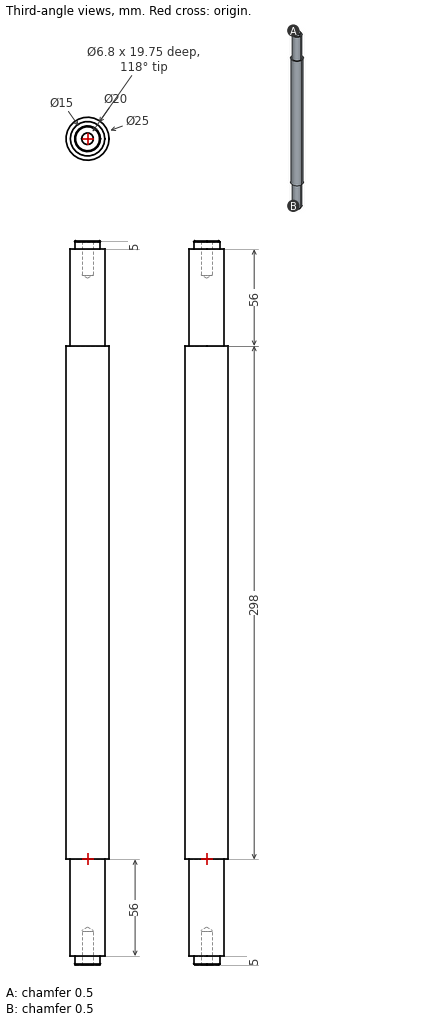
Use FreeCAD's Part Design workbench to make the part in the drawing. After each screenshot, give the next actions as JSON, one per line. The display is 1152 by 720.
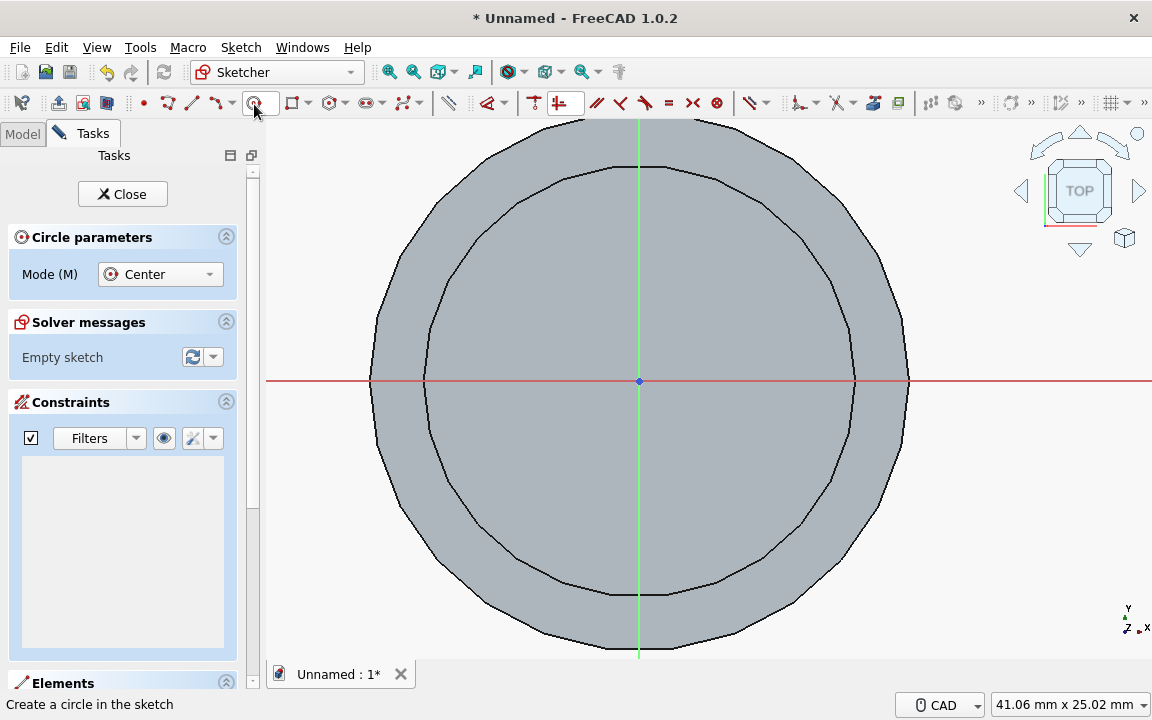
{"action": "left_click", "coordinate": [639, 381]}
{"action": "left_click", "coordinate": [754, 267]}
{"action": "key", "text": "Escape"}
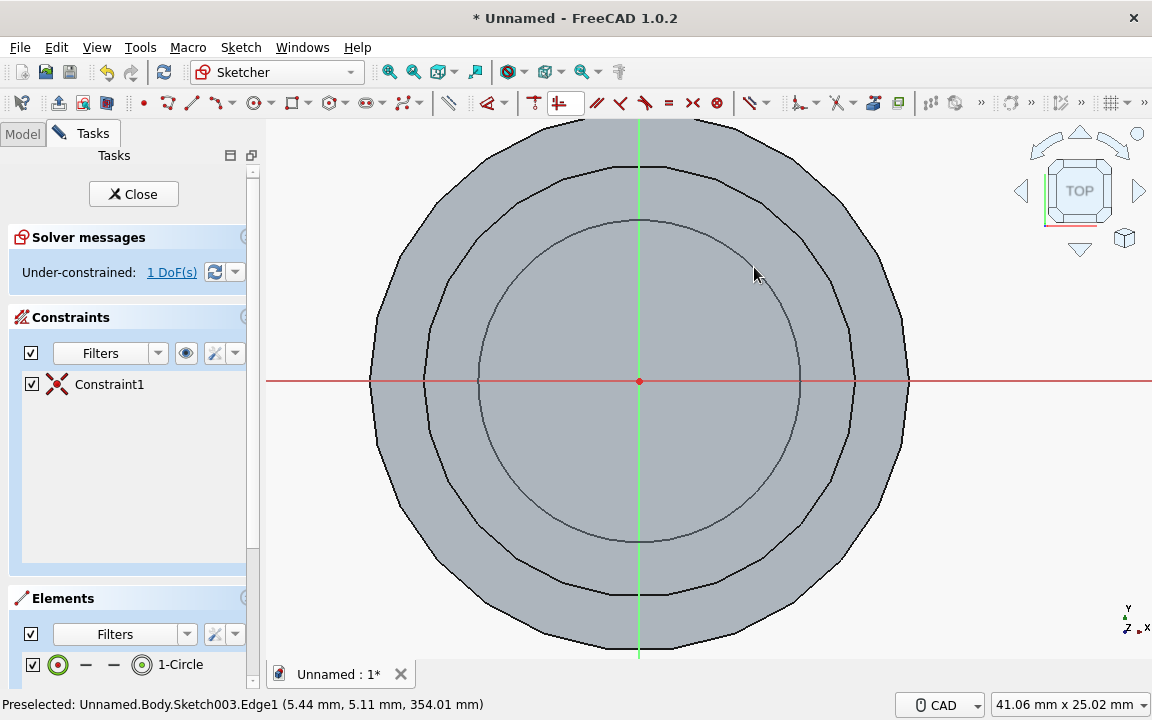
{"action": "left_click", "coordinate": [488, 104]}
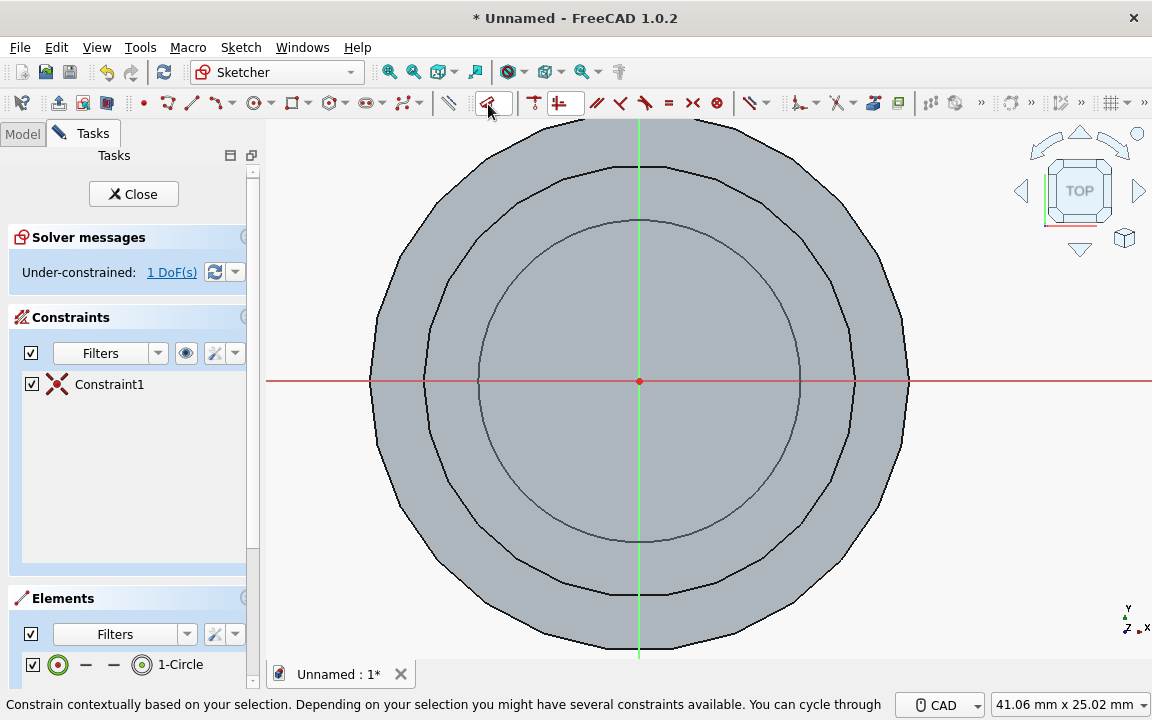
{"action": "left_click", "coordinate": [753, 267]}
{"action": "left_click", "coordinate": [776, 244]}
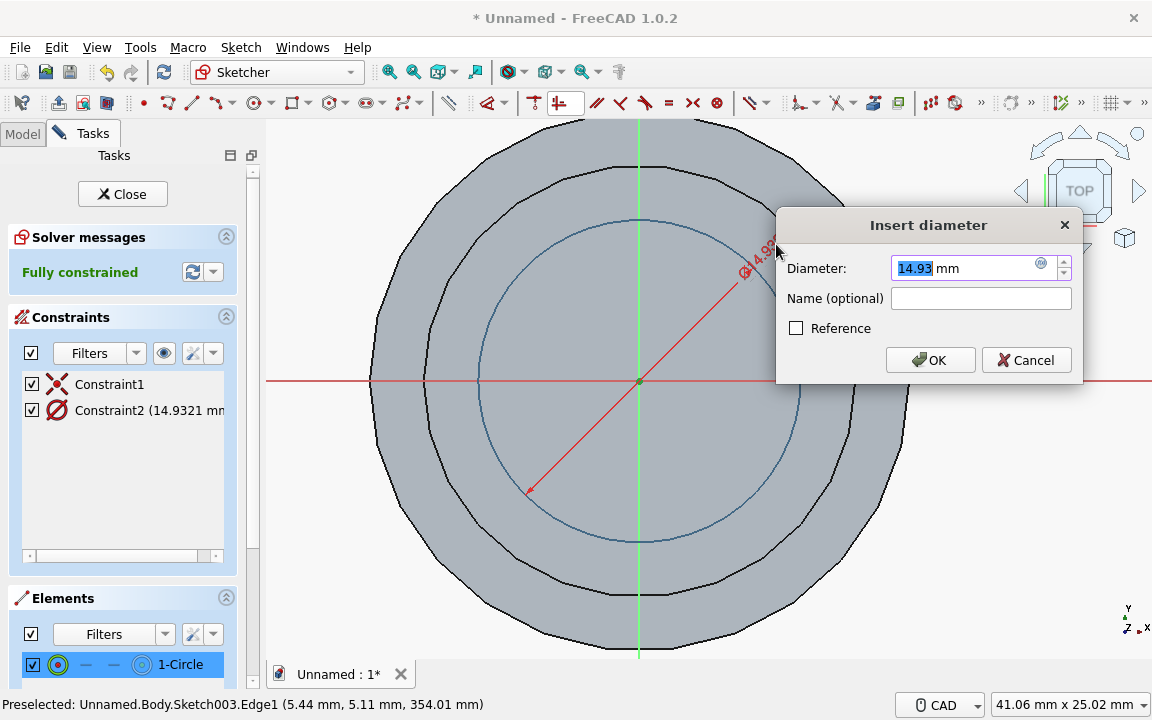
{"action": "type", "text": "15"}
{"action": "key", "text": "Return"}
{"action": "key", "text": "Escape"}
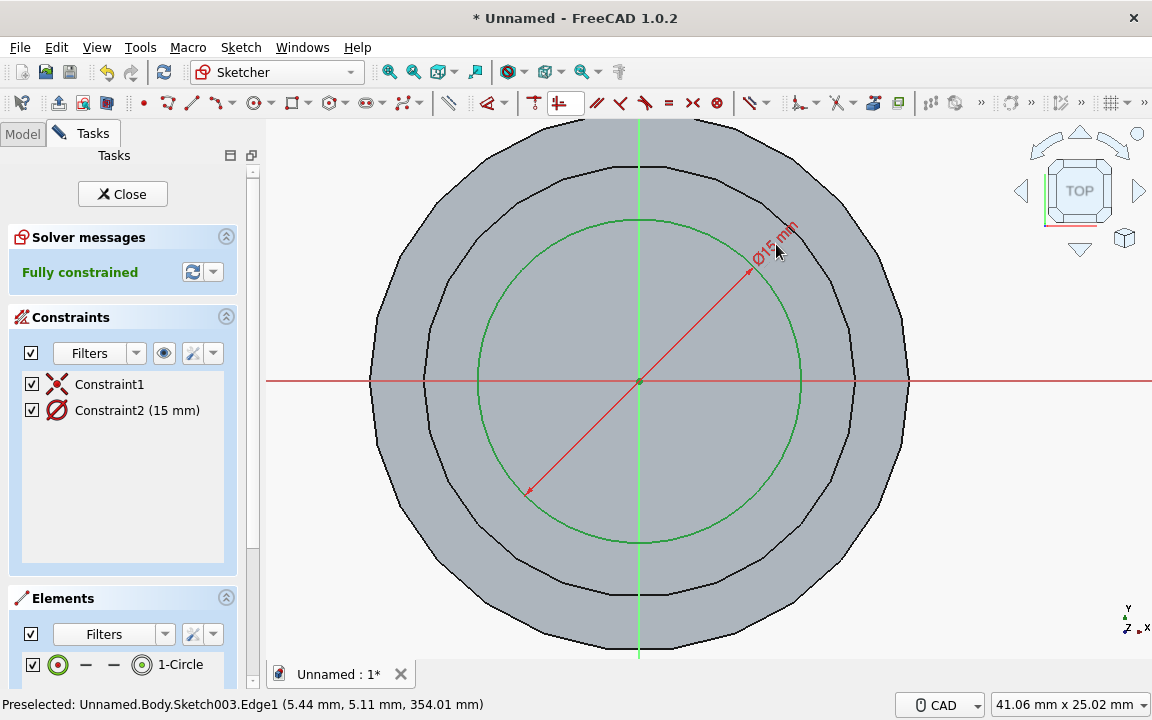
{"action": "left_click", "coordinate": [123, 194]}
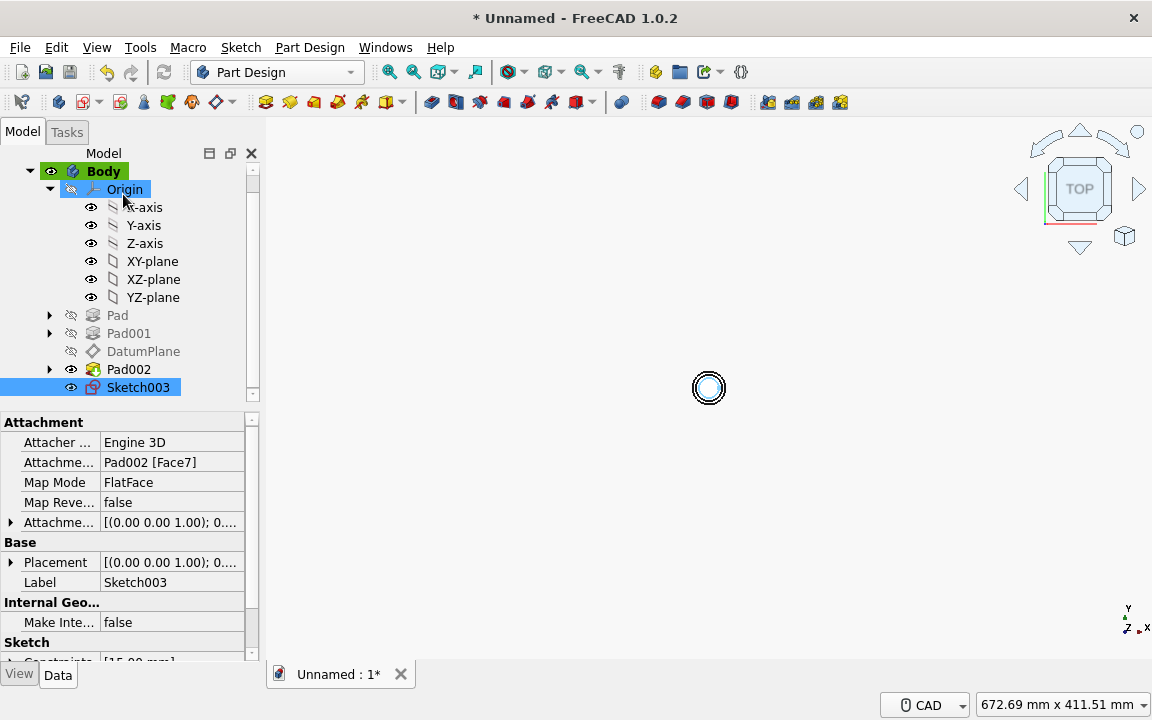
{"action": "left_click", "coordinate": [266, 102]}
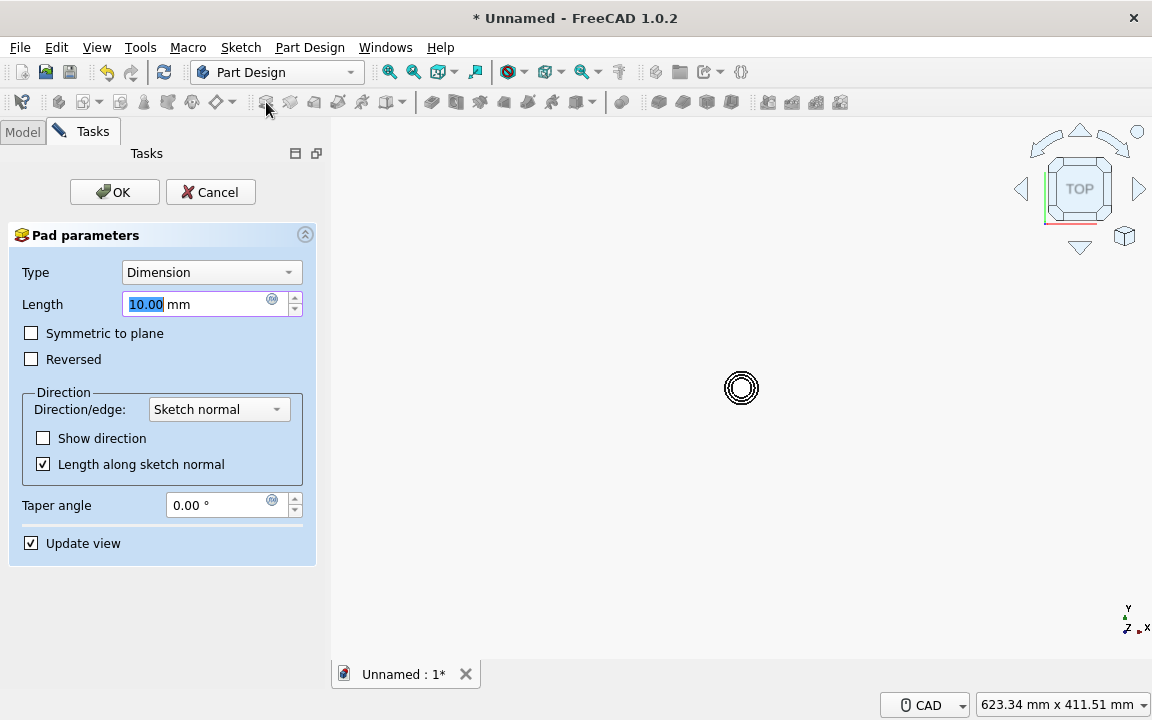
{"action": "type", "text": "5"}
{"action": "key", "text": "Tab"}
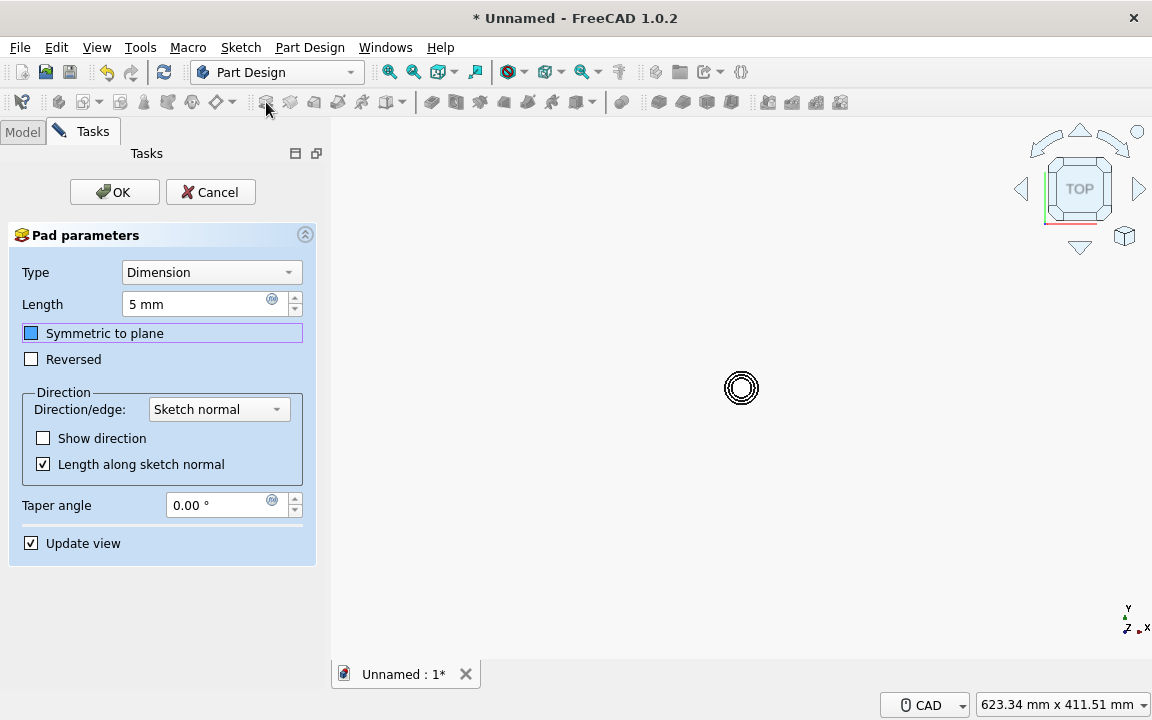
{"action": "left_click", "coordinate": [115, 192]}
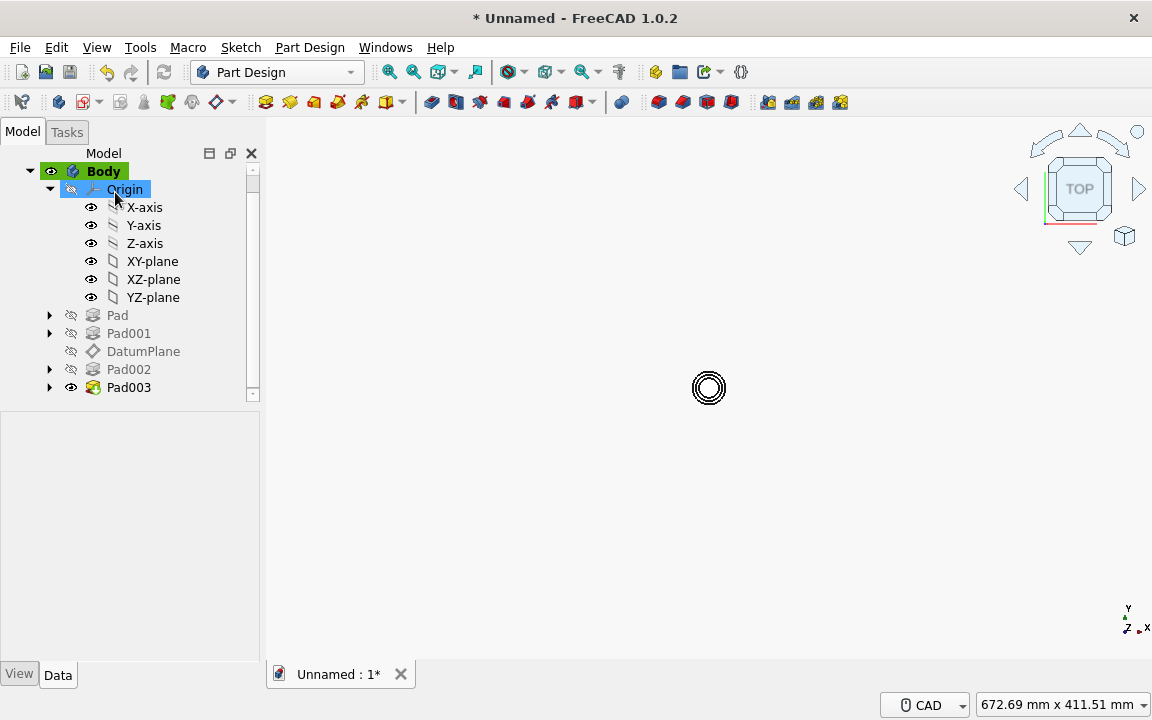
{"action": "left_click", "coordinate": [390, 72]}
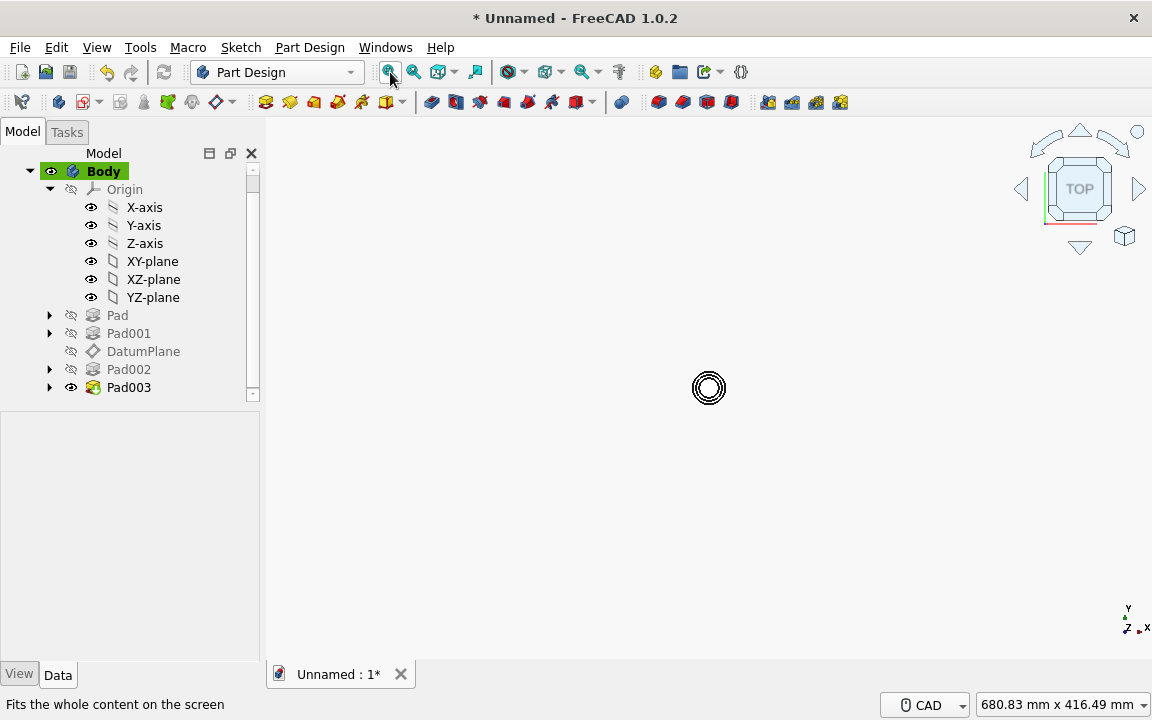
{"action": "left_click", "coordinate": [136, 261]}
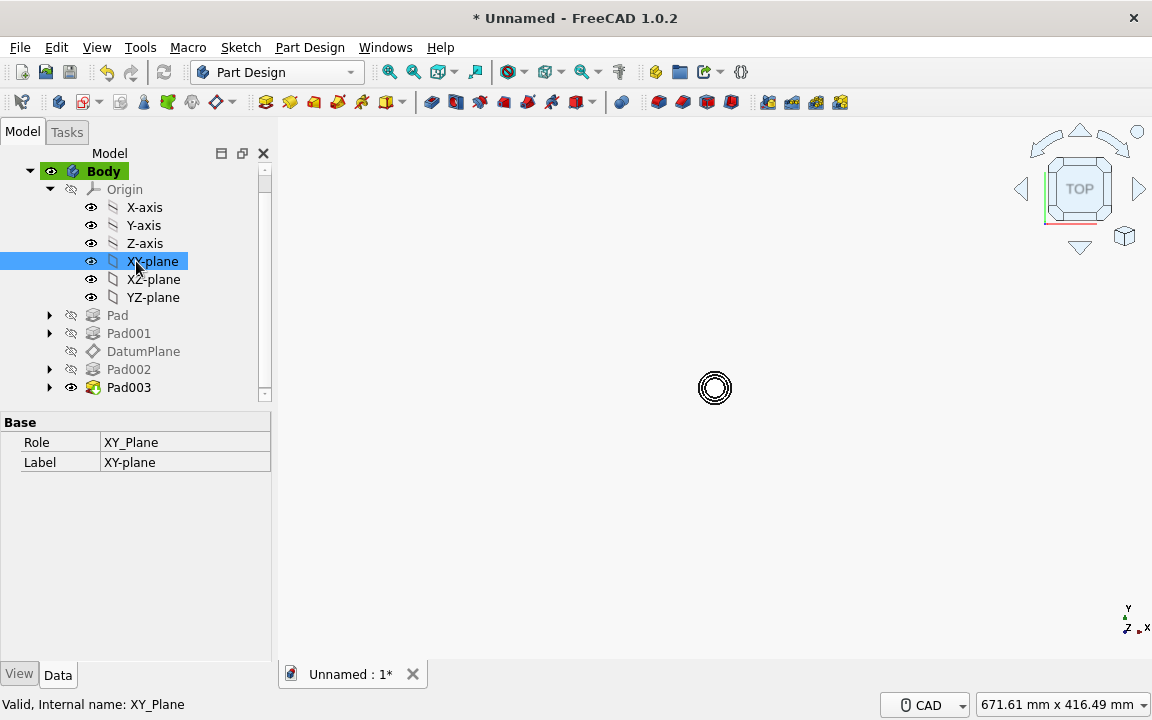
{"action": "left_click", "coordinate": [216, 102]}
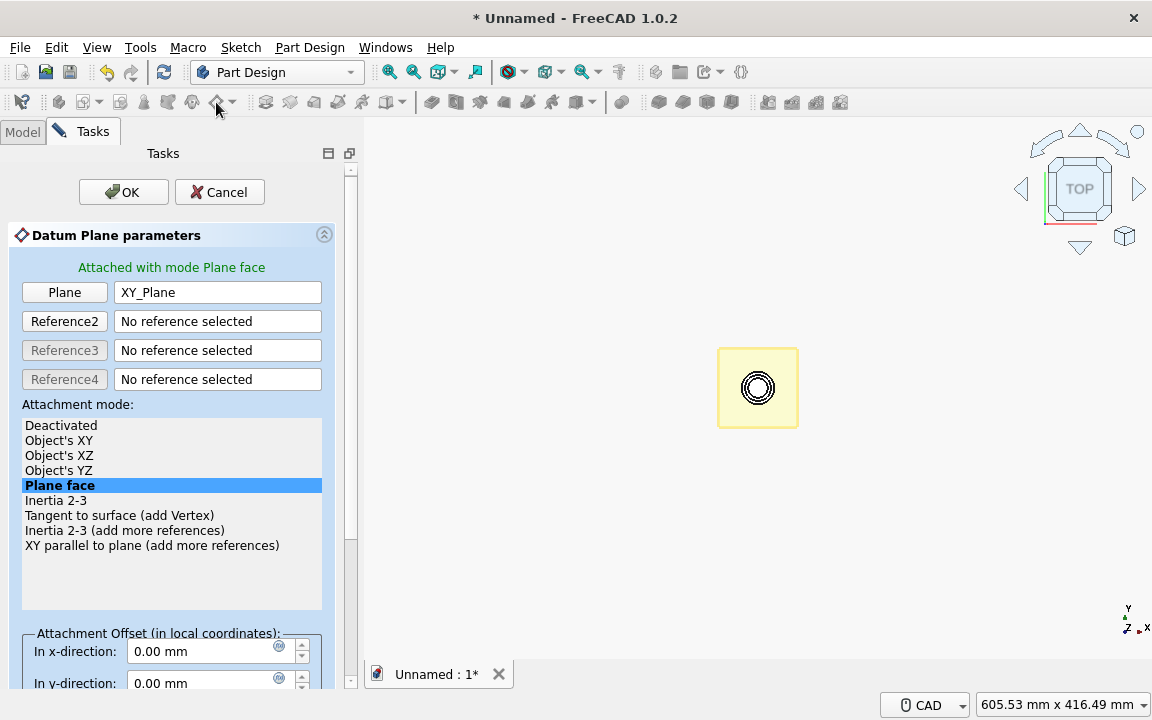
{"action": "scroll", "coordinate": [351, 426], "scroll_direction": "down", "scroll_amount": 2}